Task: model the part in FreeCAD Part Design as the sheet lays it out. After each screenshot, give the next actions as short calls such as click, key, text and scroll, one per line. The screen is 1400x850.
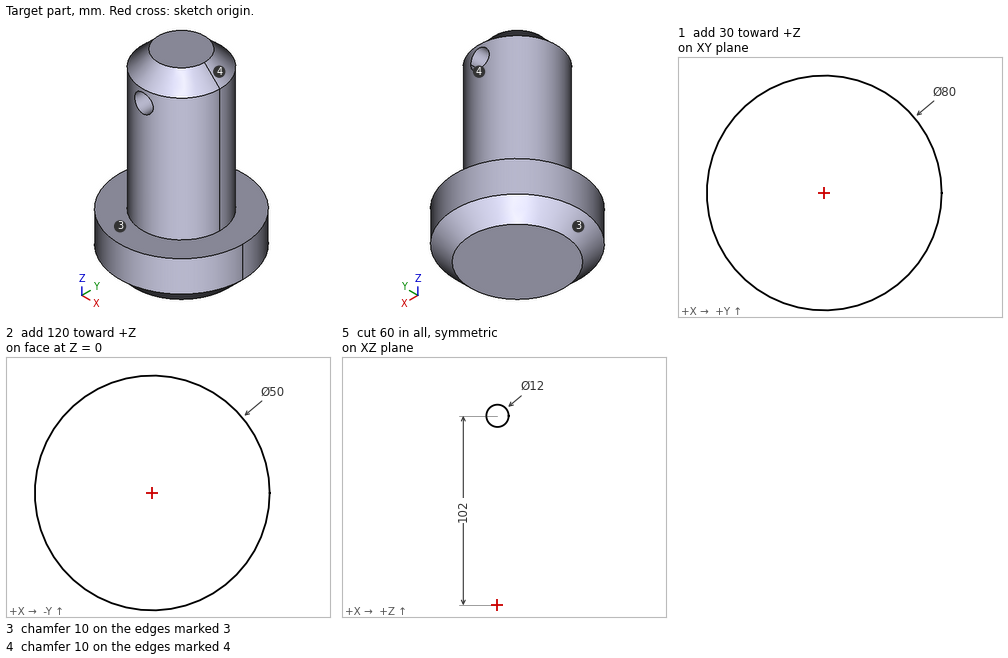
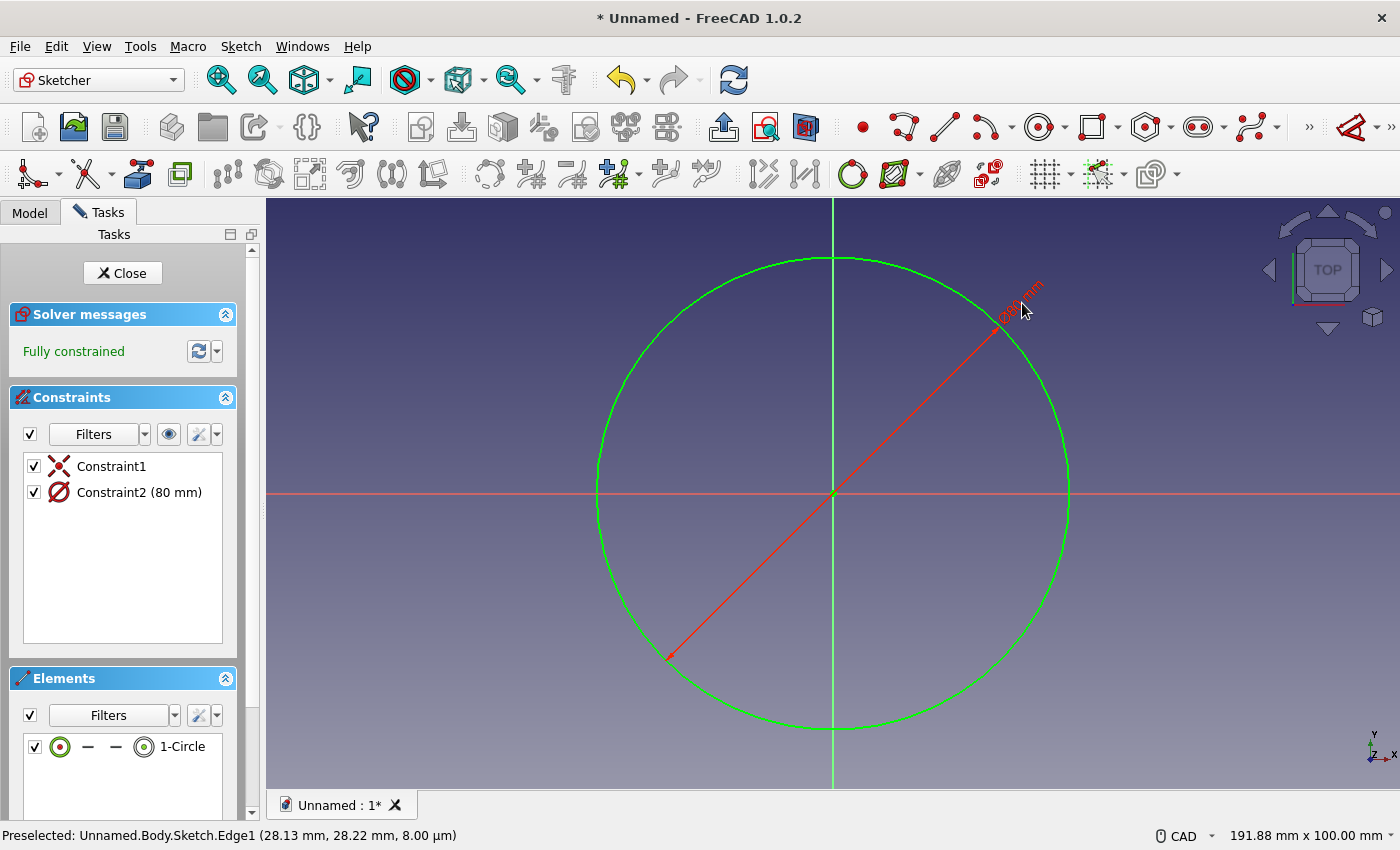
click(123, 273)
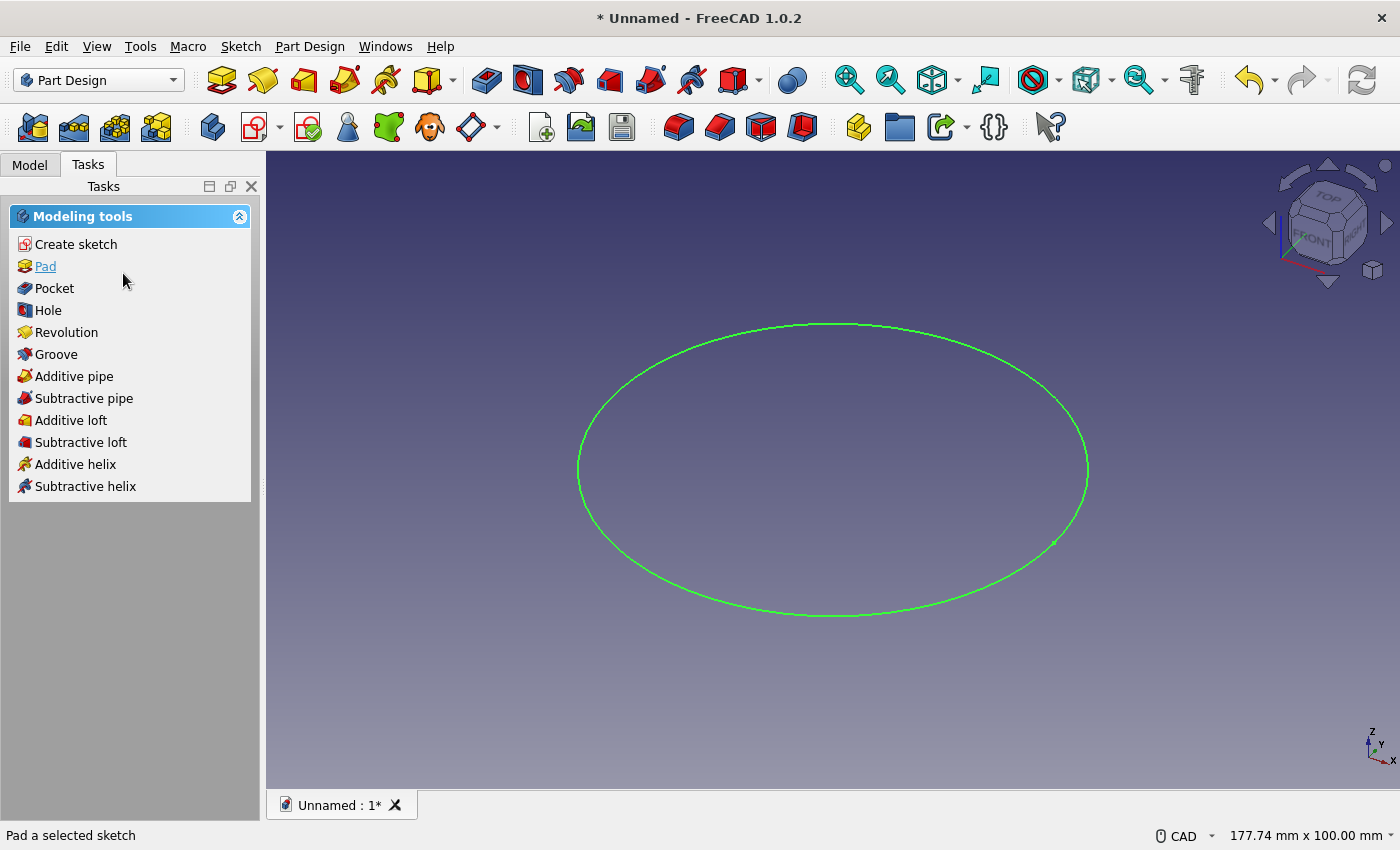
click(222, 80)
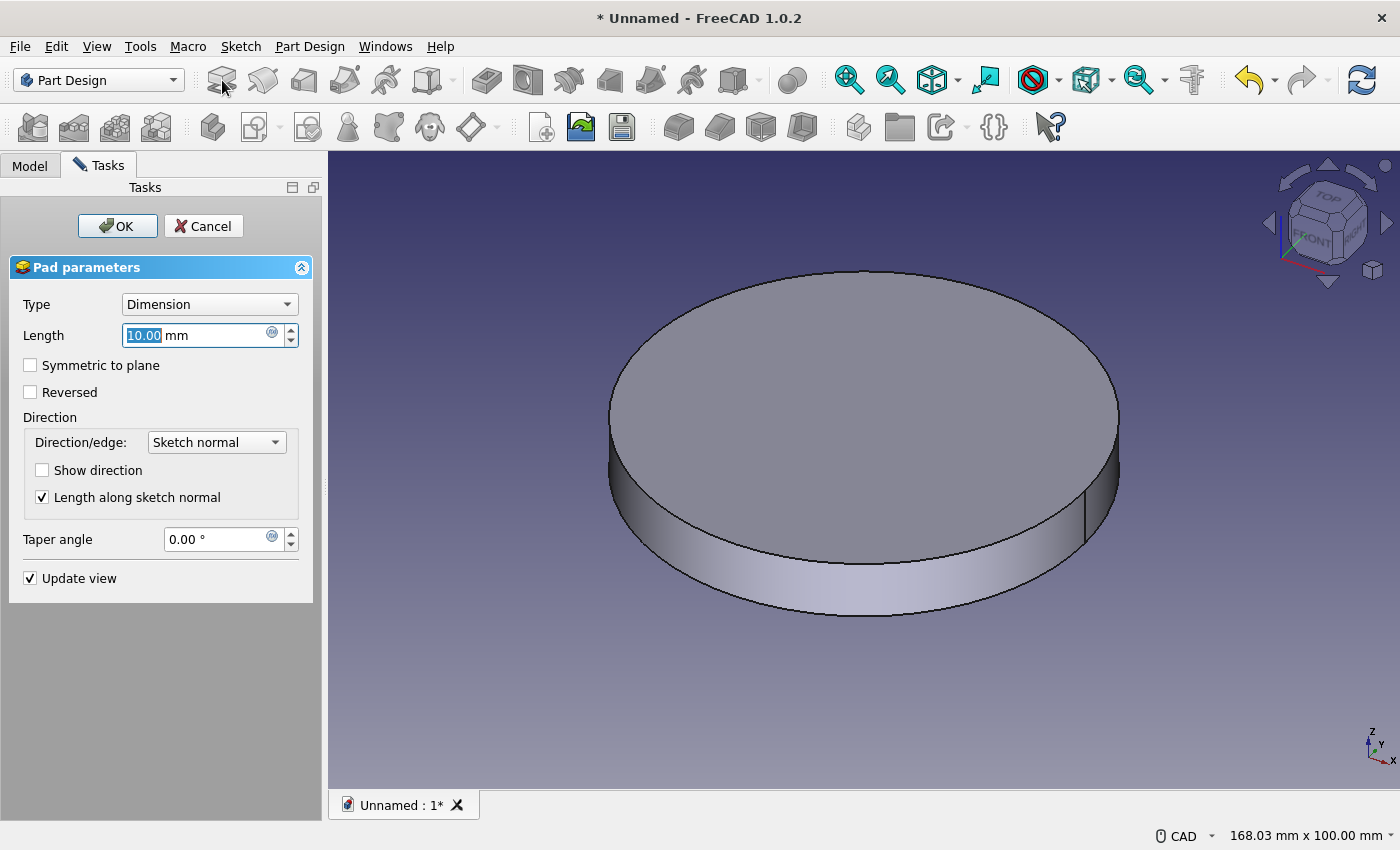
text(30)
key(Tab)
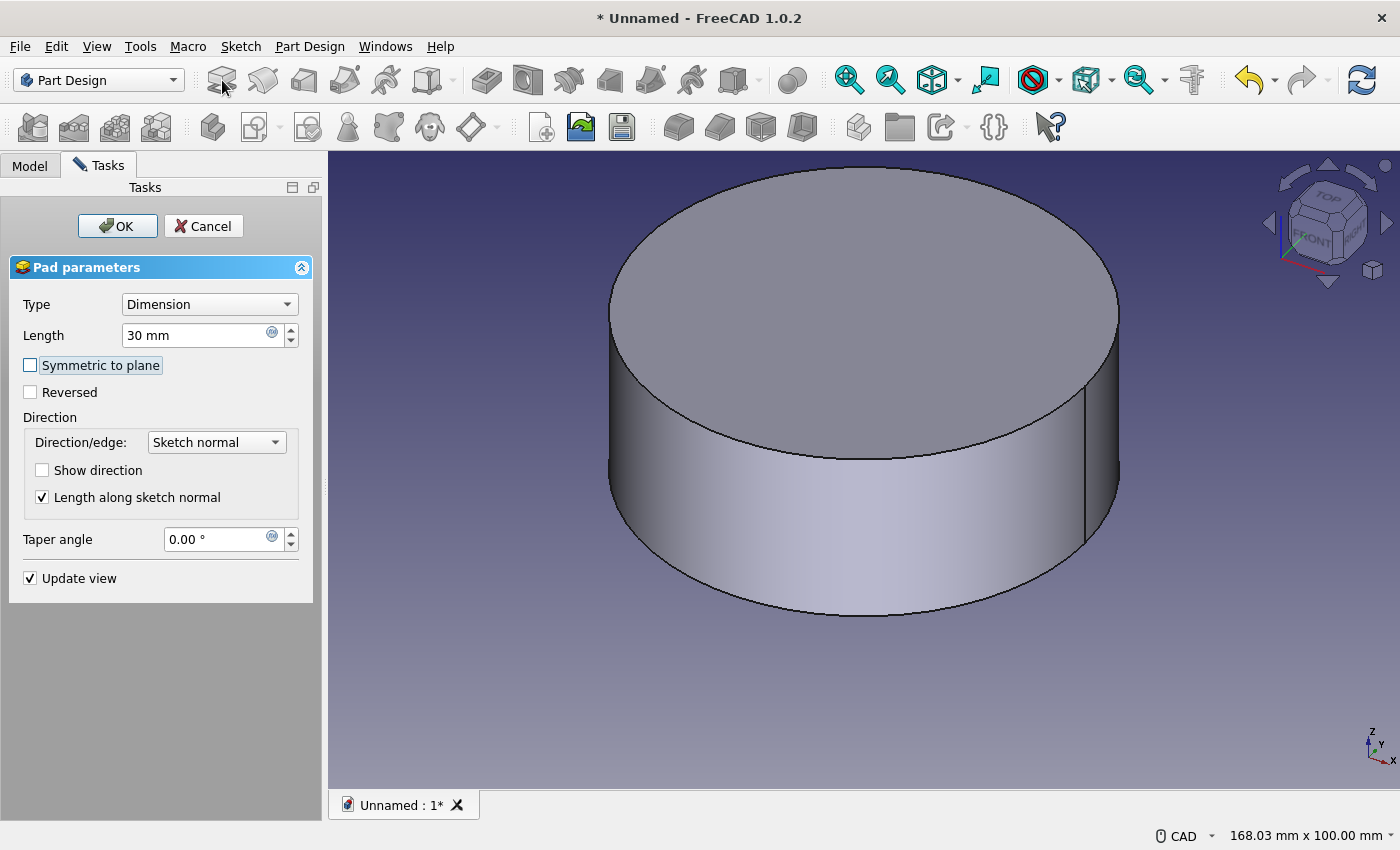
click(118, 226)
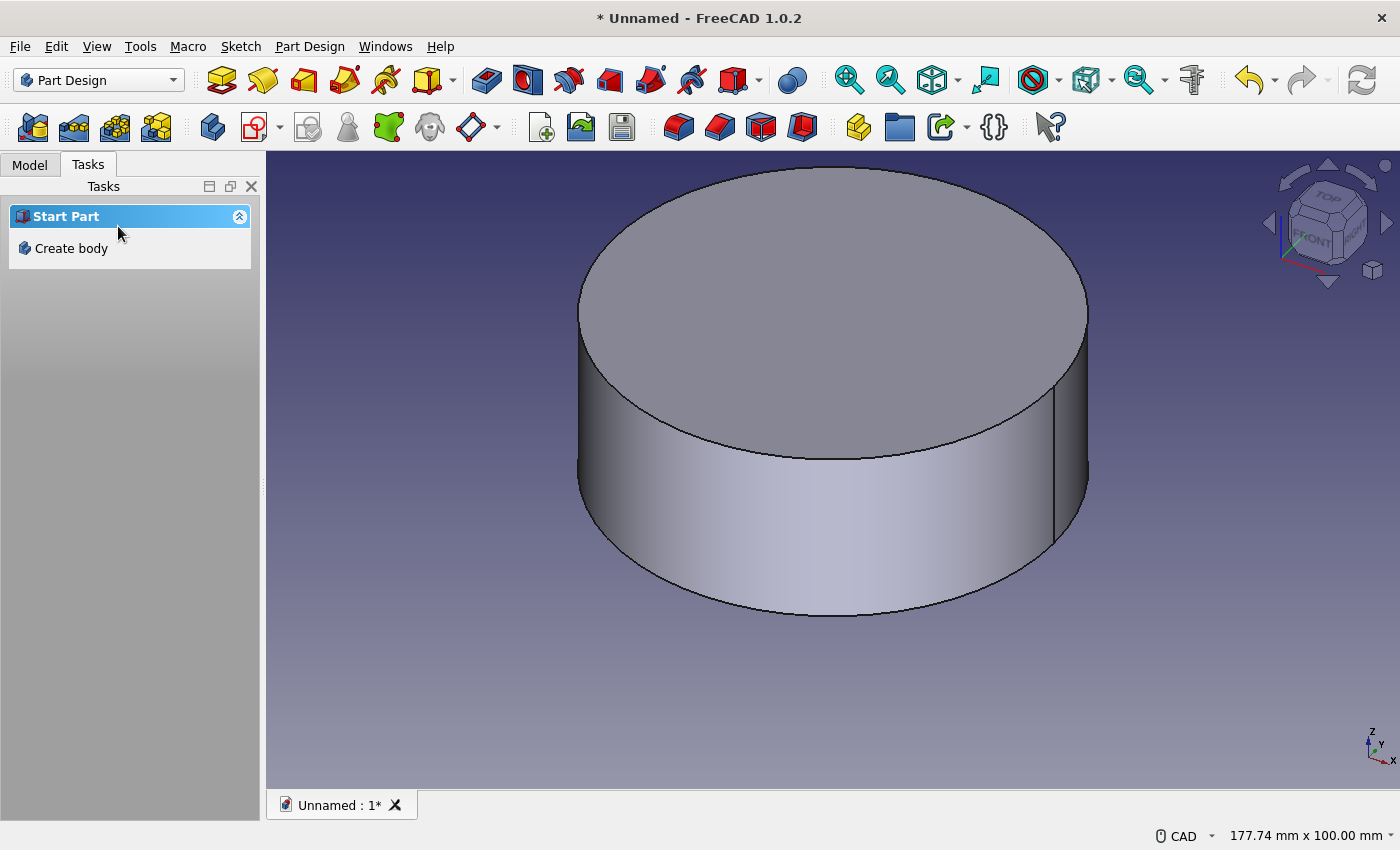
key(v)
key(f)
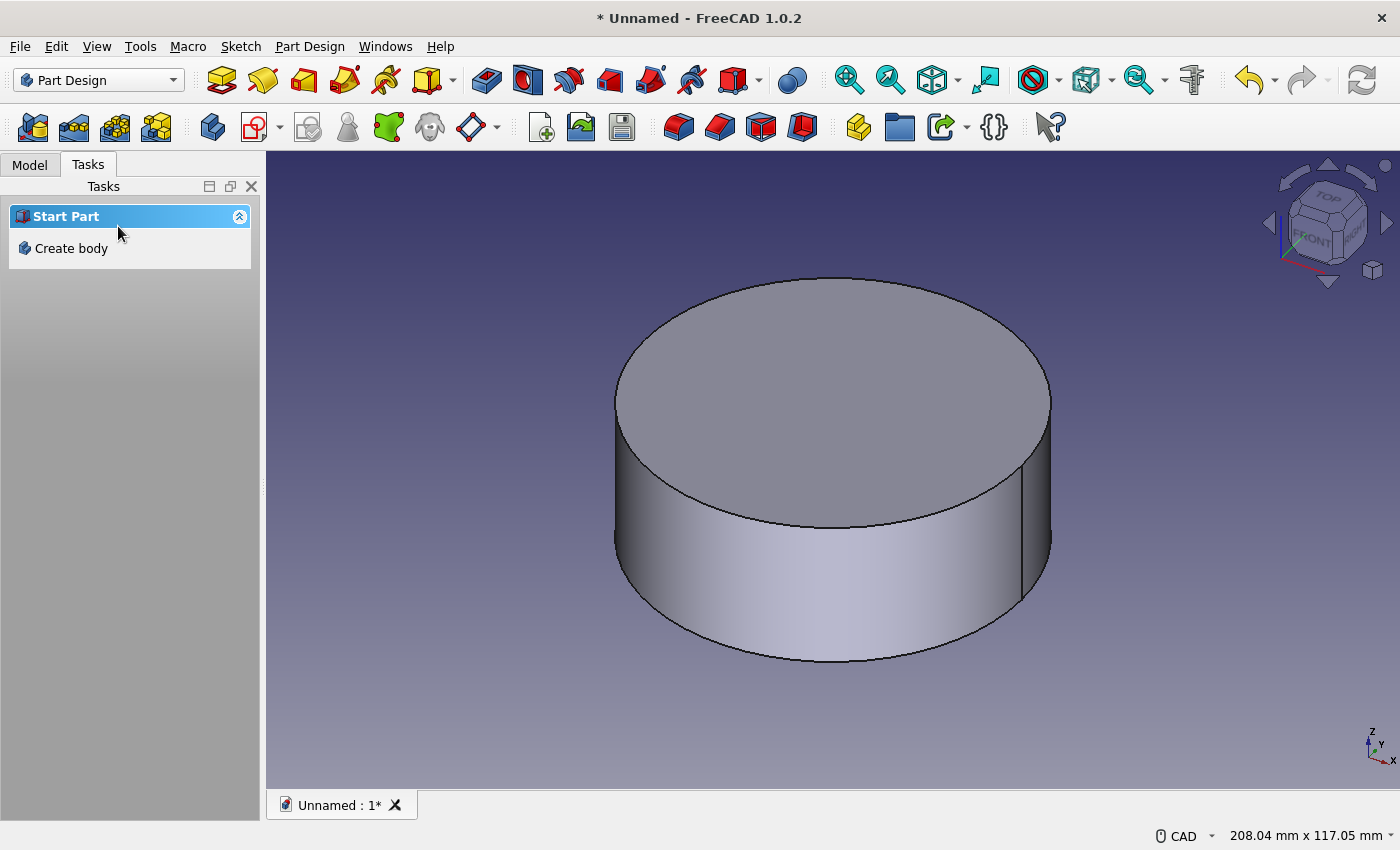
key(5)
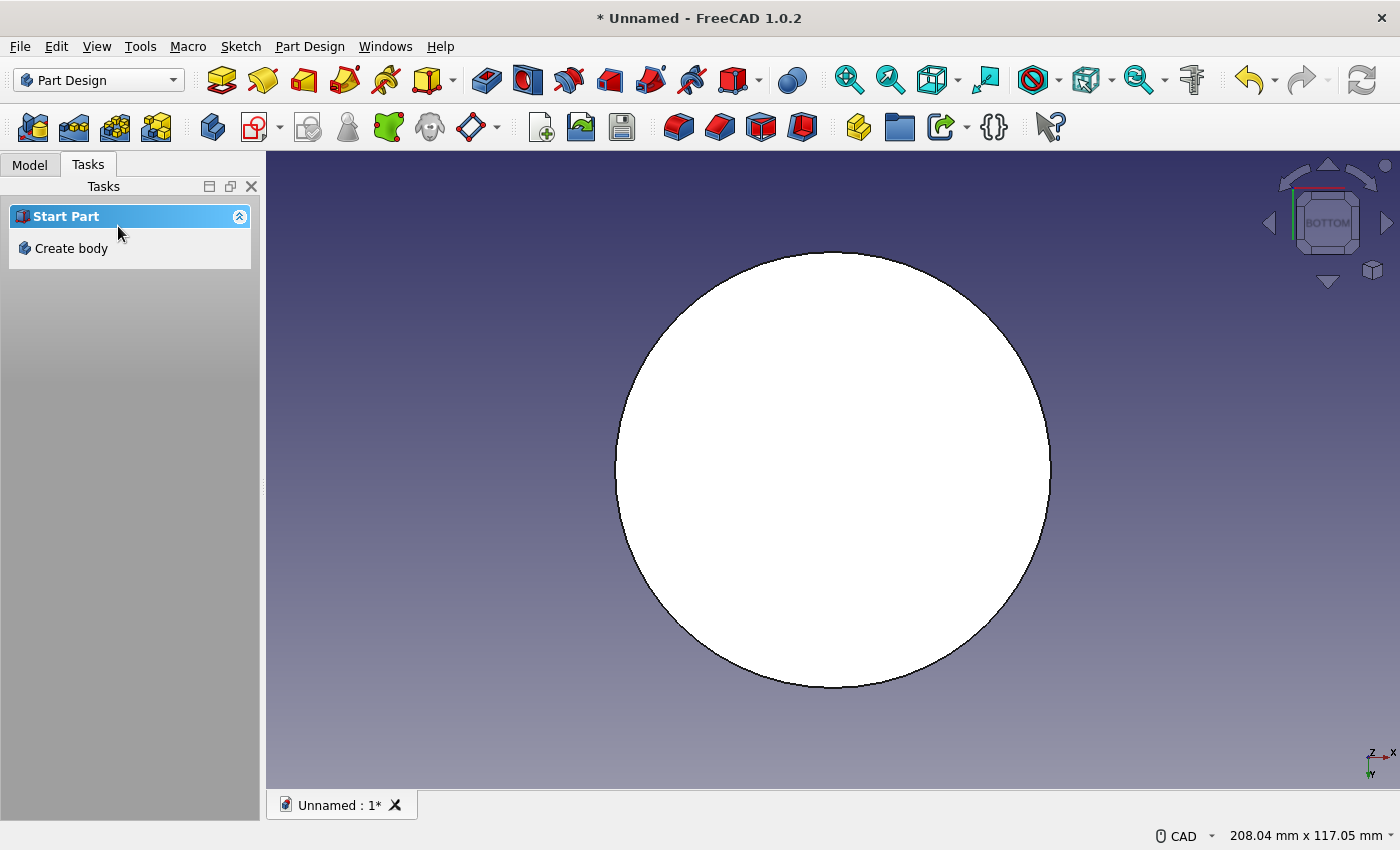
click(833, 469)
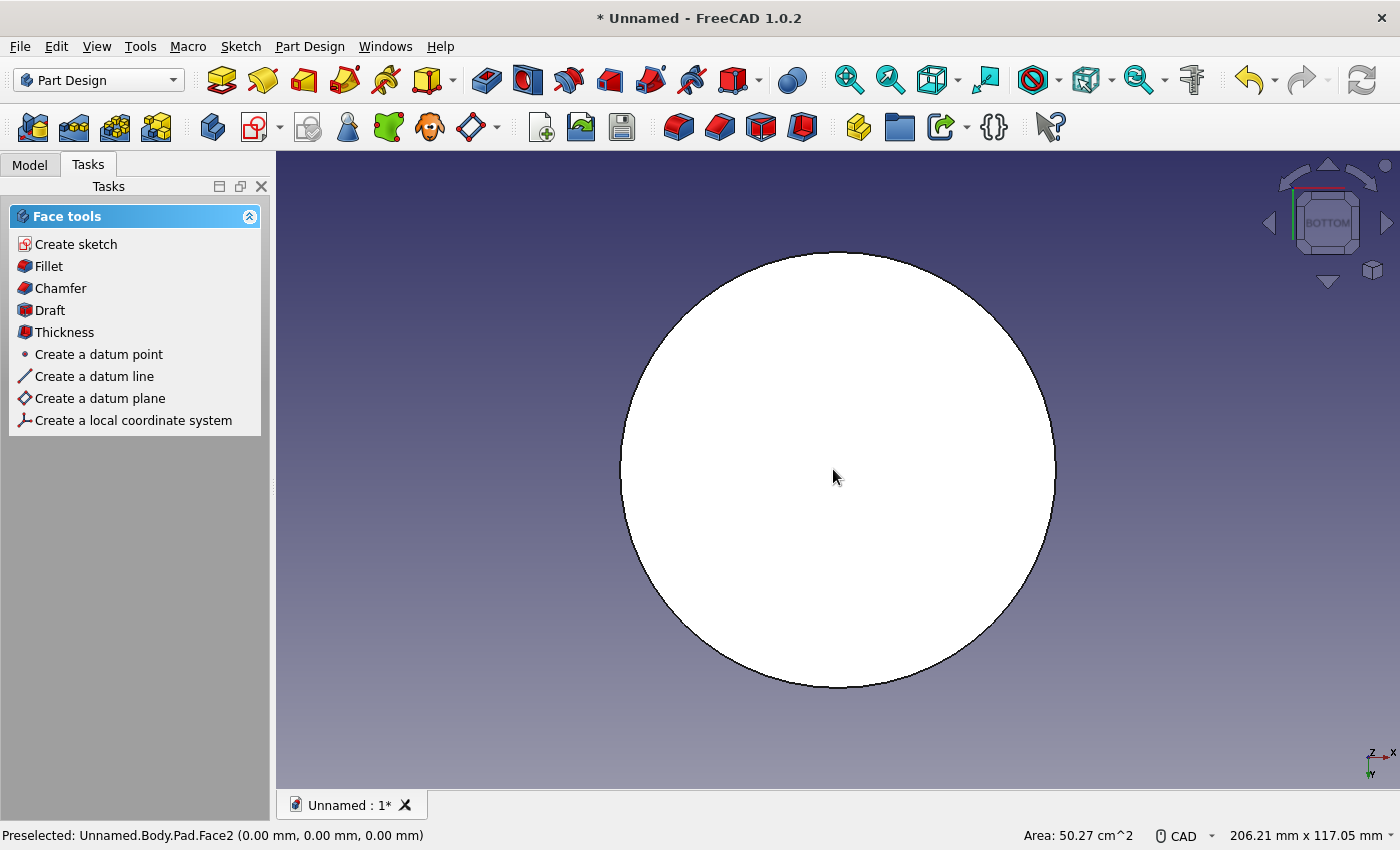
click(254, 128)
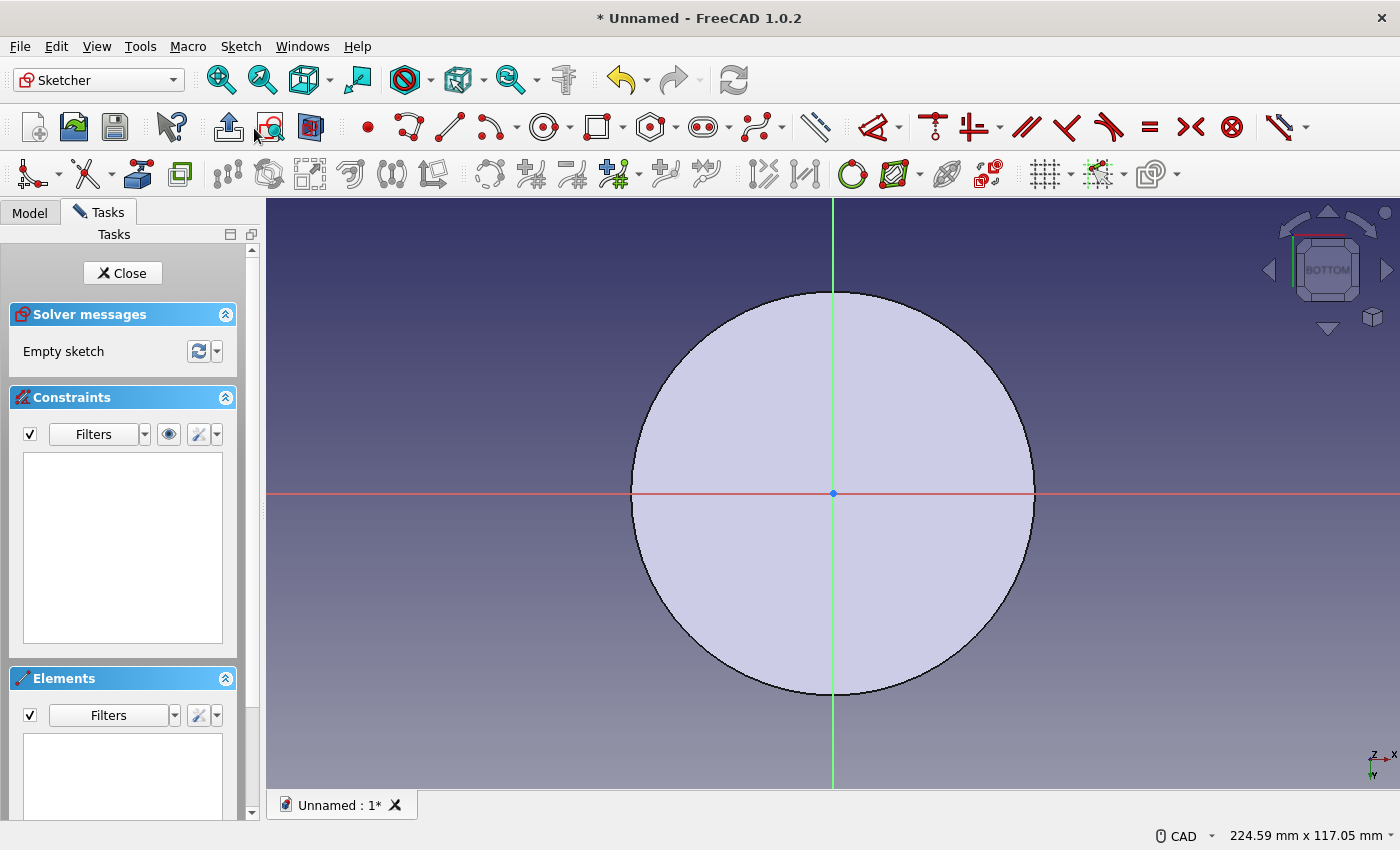
scroll(972, 493, up, 2)